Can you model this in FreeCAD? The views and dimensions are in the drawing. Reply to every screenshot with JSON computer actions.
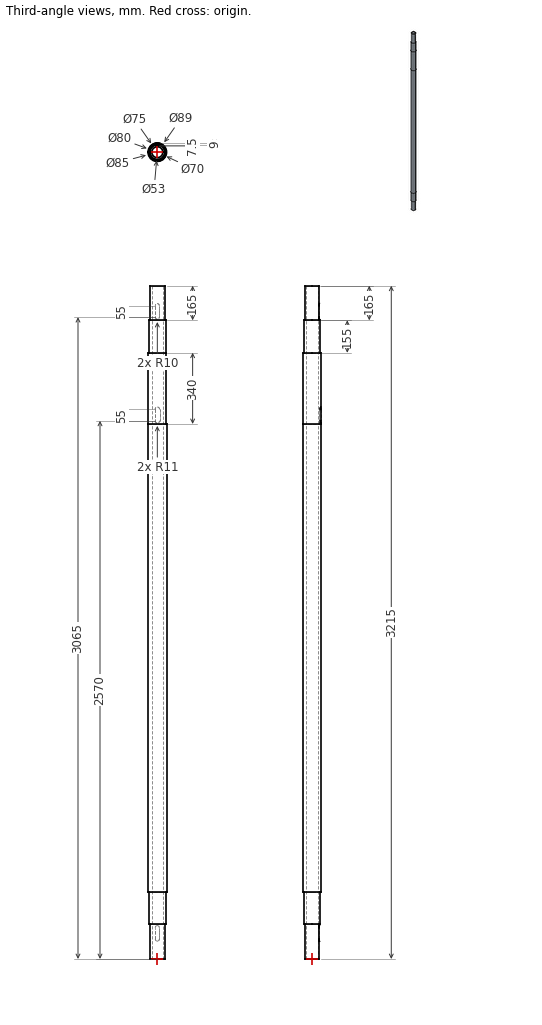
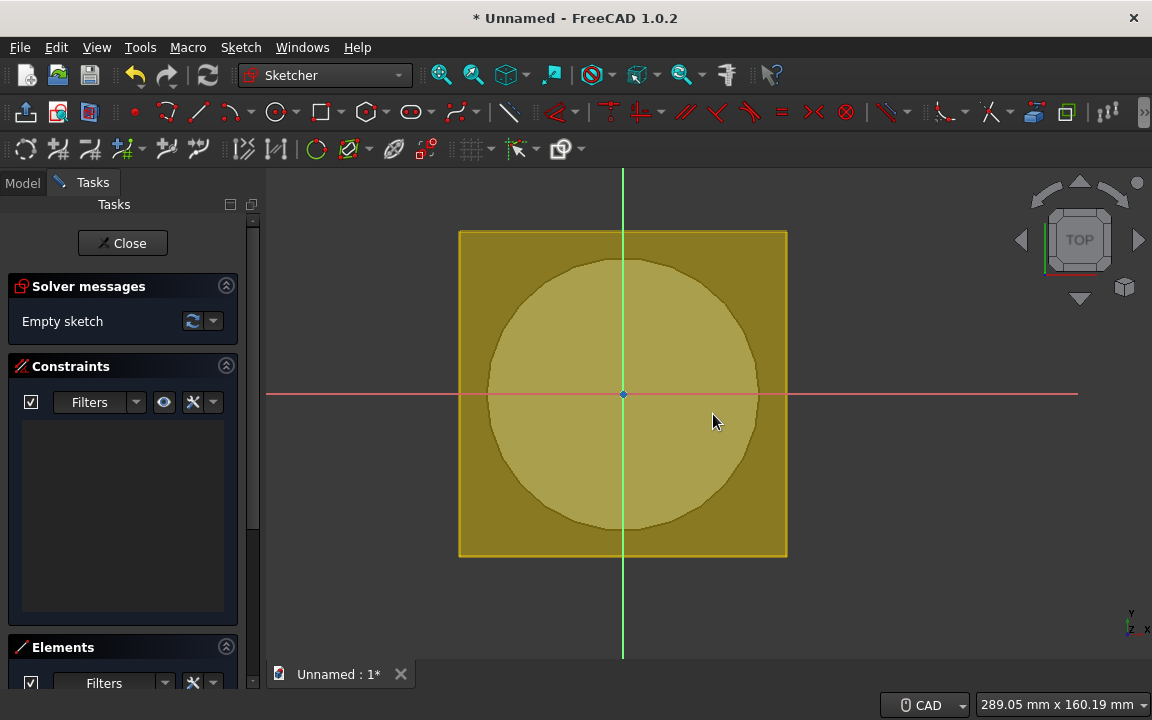
{"action": "left_click", "coordinate": [276, 112]}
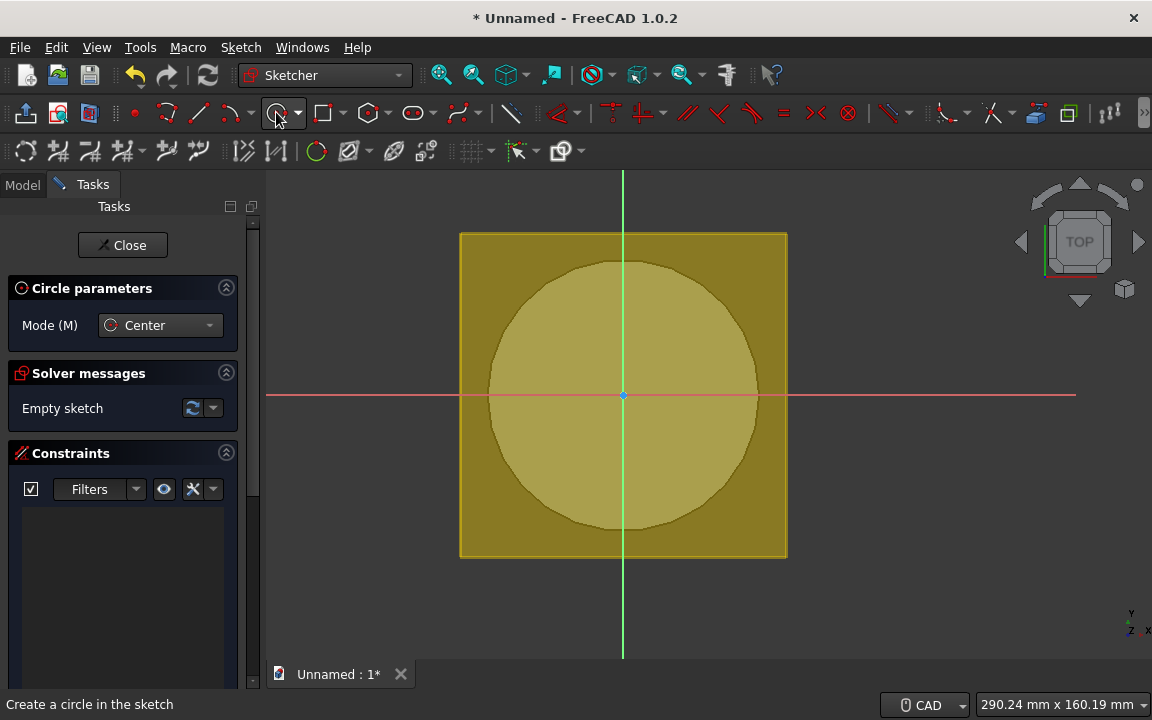
{"action": "left_click", "coordinate": [623, 395]}
{"action": "mouse_move", "coordinate": [719, 299]}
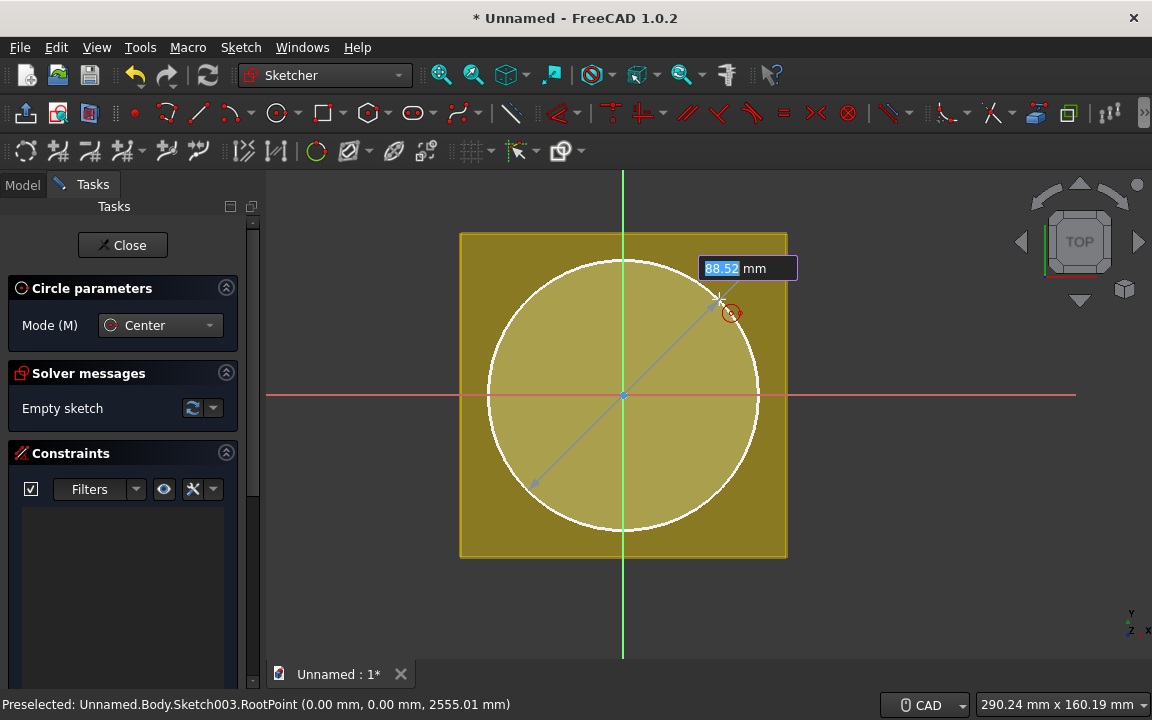
{"action": "type", "text": "89"}
{"action": "key", "text": "Return"}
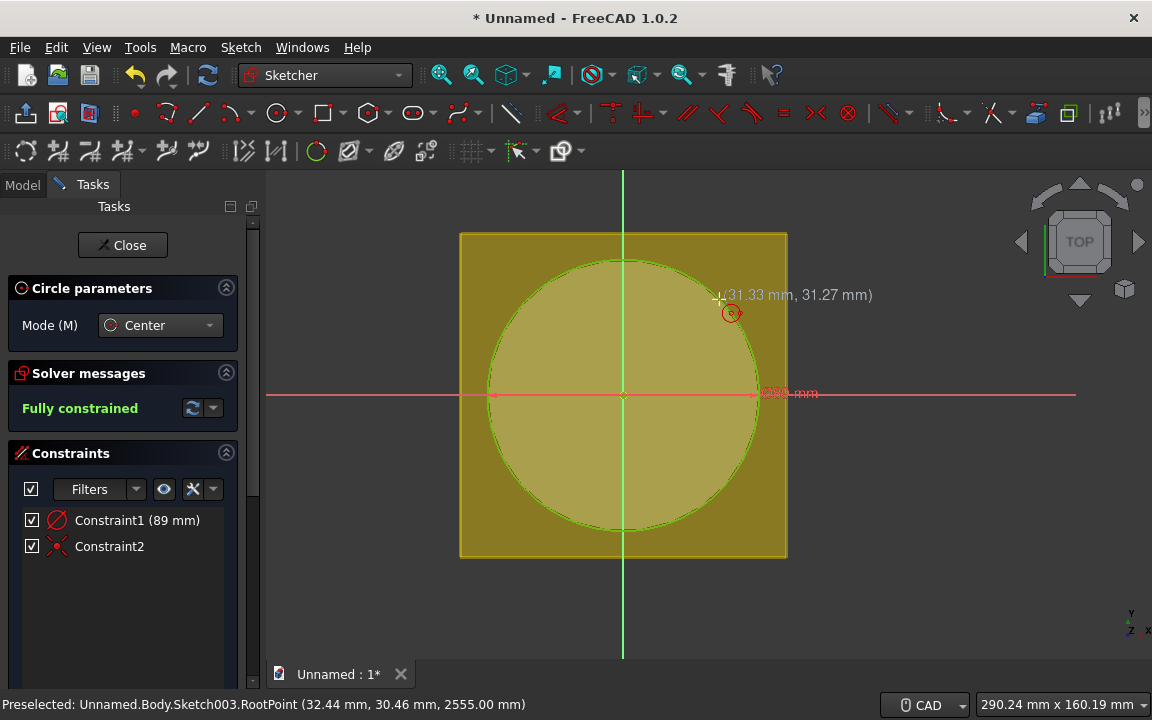
{"action": "left_click", "coordinate": [623, 395]}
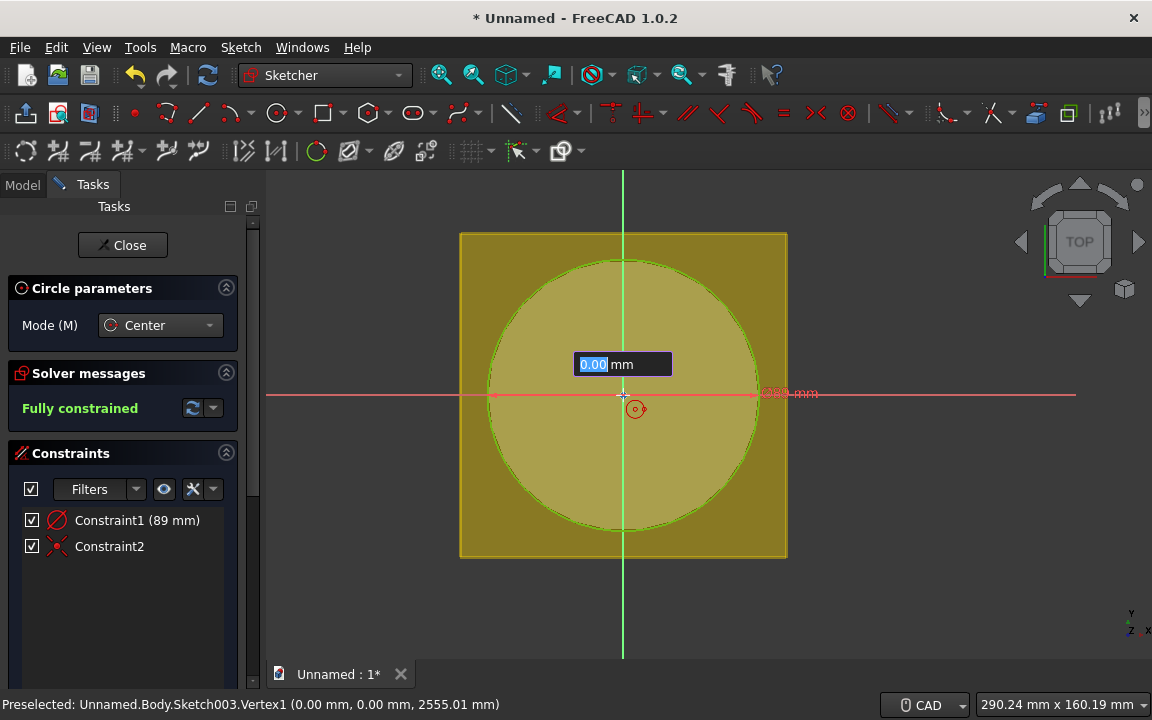
{"action": "scroll", "coordinate": [715, 304], "scroll_direction": "up", "scroll_amount": 5}
{"action": "mouse_move", "coordinate": [714, 303]}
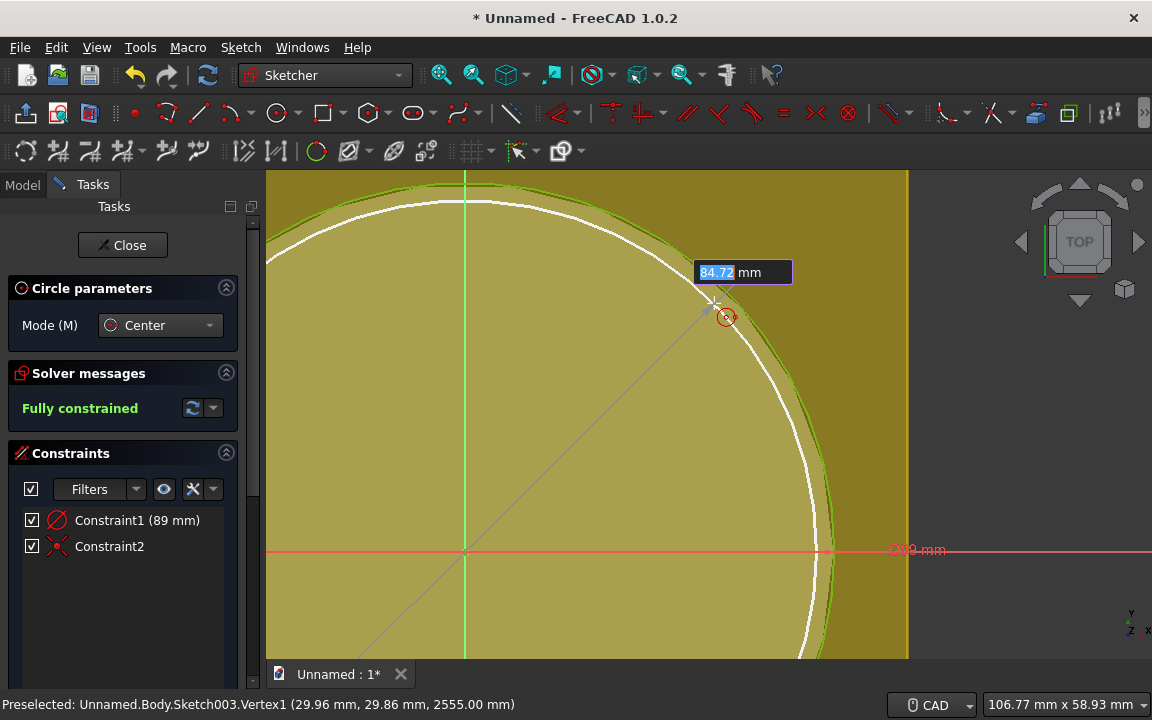
{"action": "type", "text": "85"}
{"action": "key", "text": "Return"}
{"action": "key", "text": "Escape"}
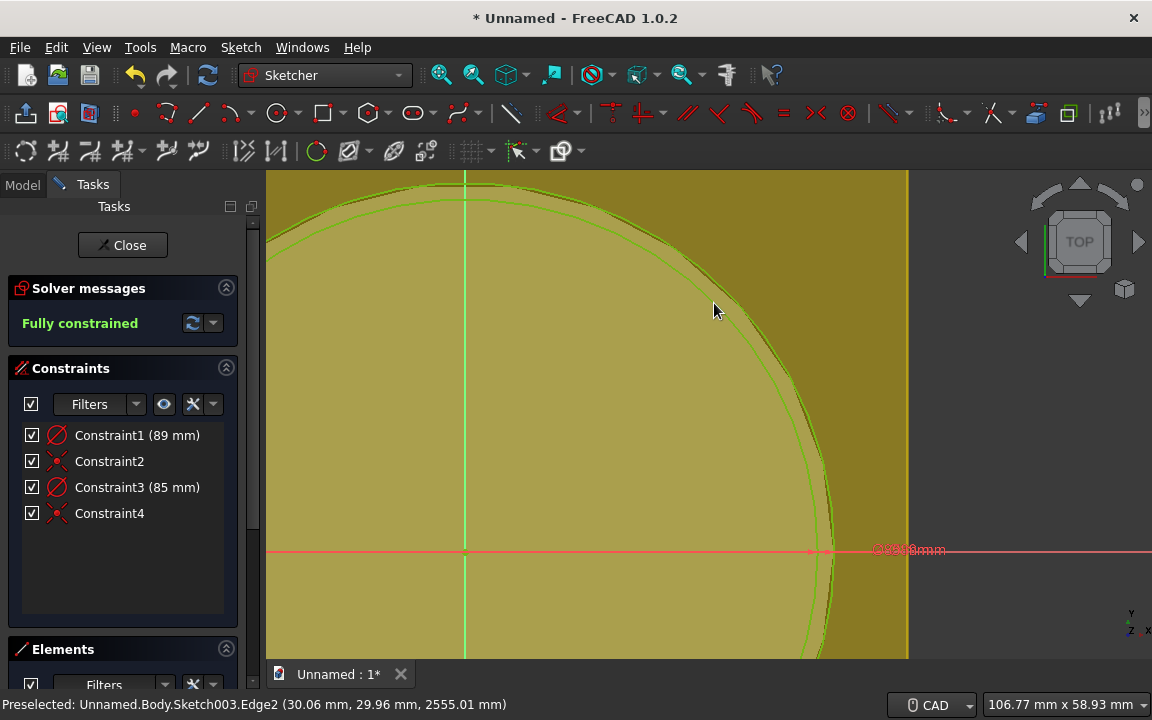
{"action": "left_click", "coordinate": [123, 245]}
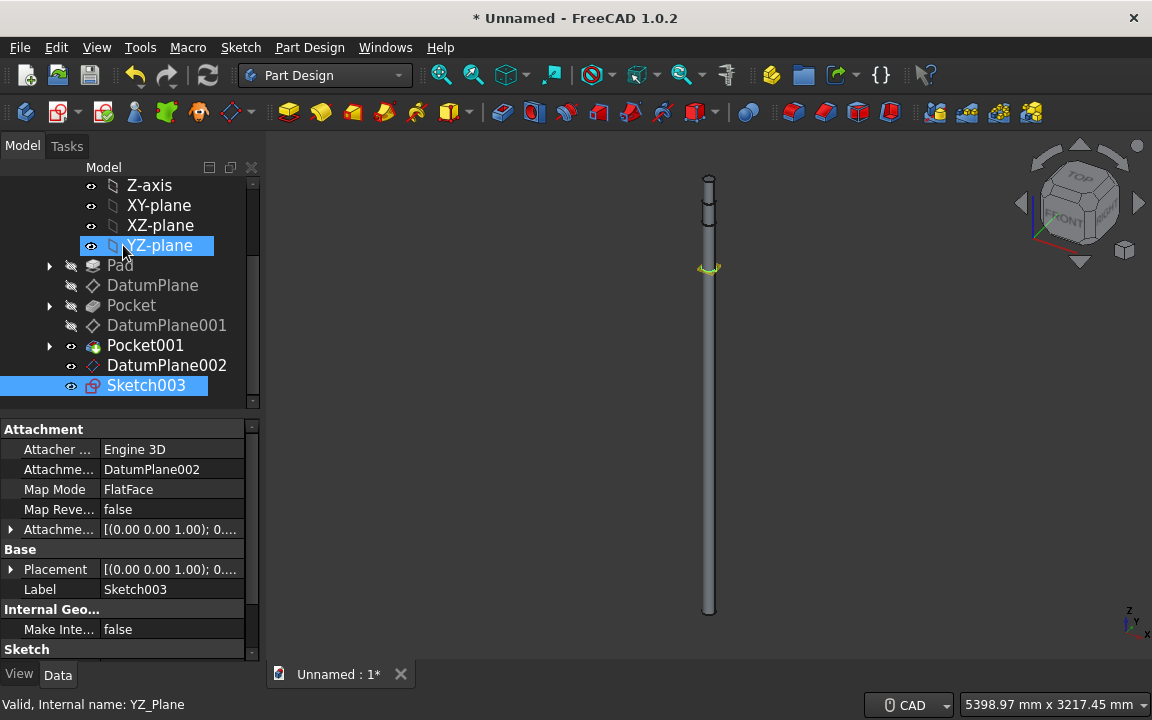
{"action": "left_click", "coordinate": [504, 112]}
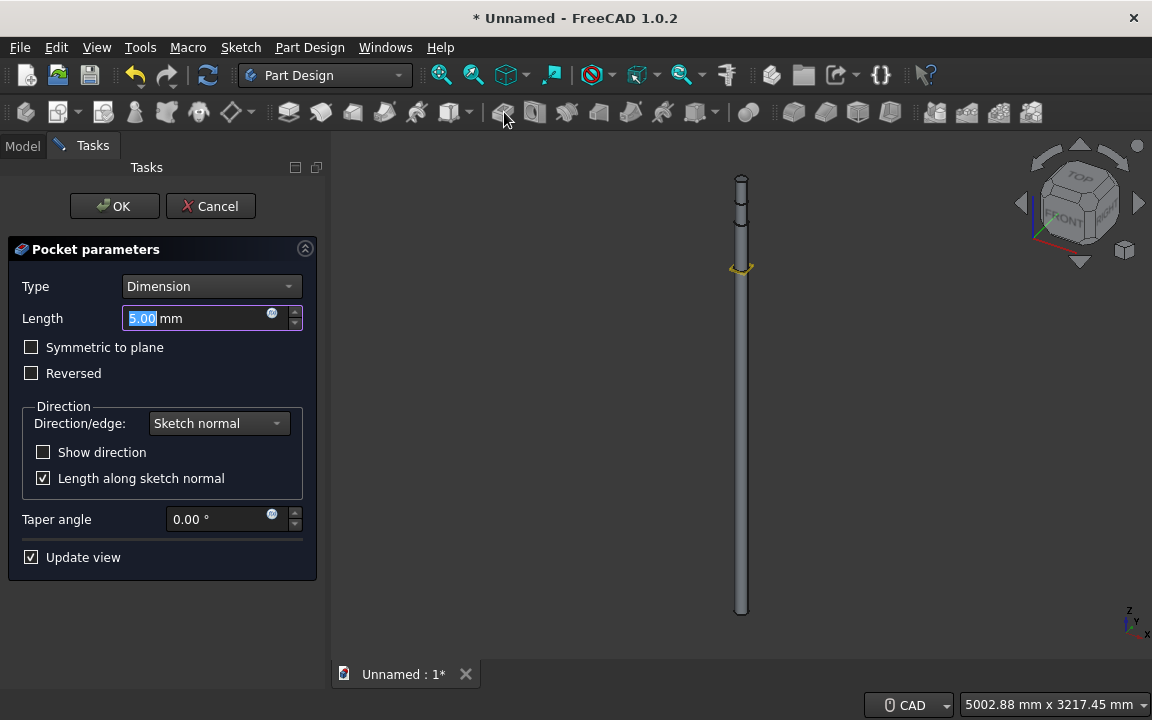
{"action": "type", "text": "340"}
{"action": "key", "text": "Tab"}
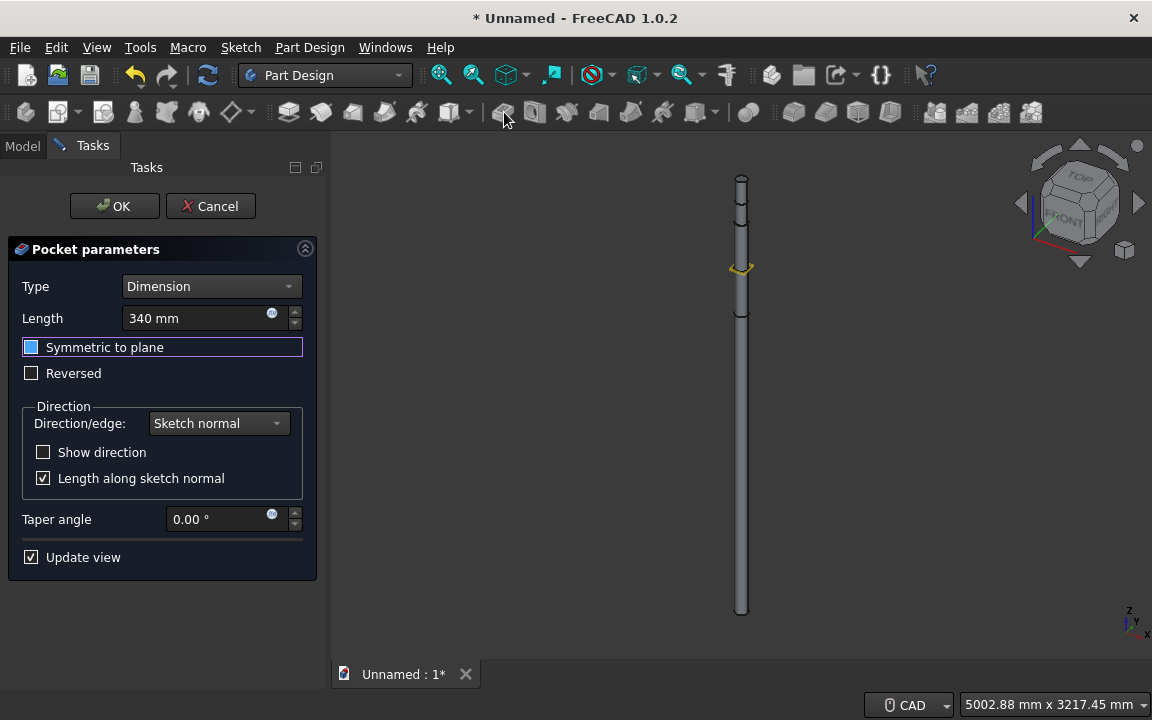
{"action": "left_click", "coordinate": [30, 373]}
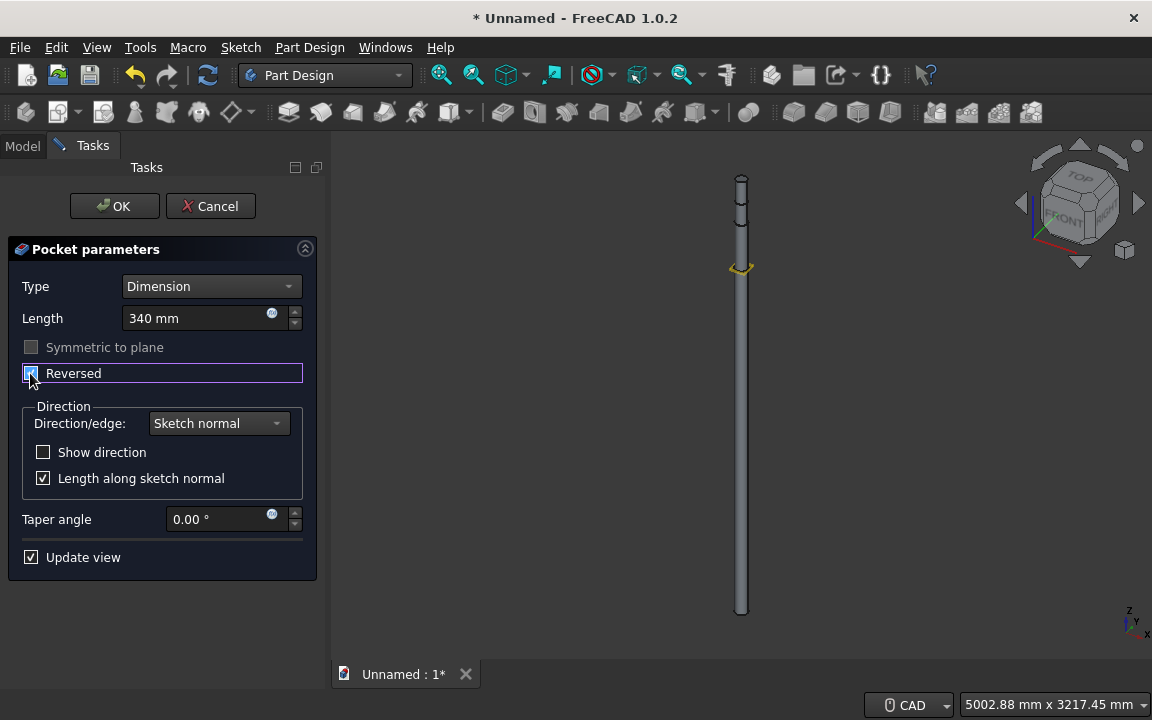
{"action": "left_click", "coordinate": [115, 206]}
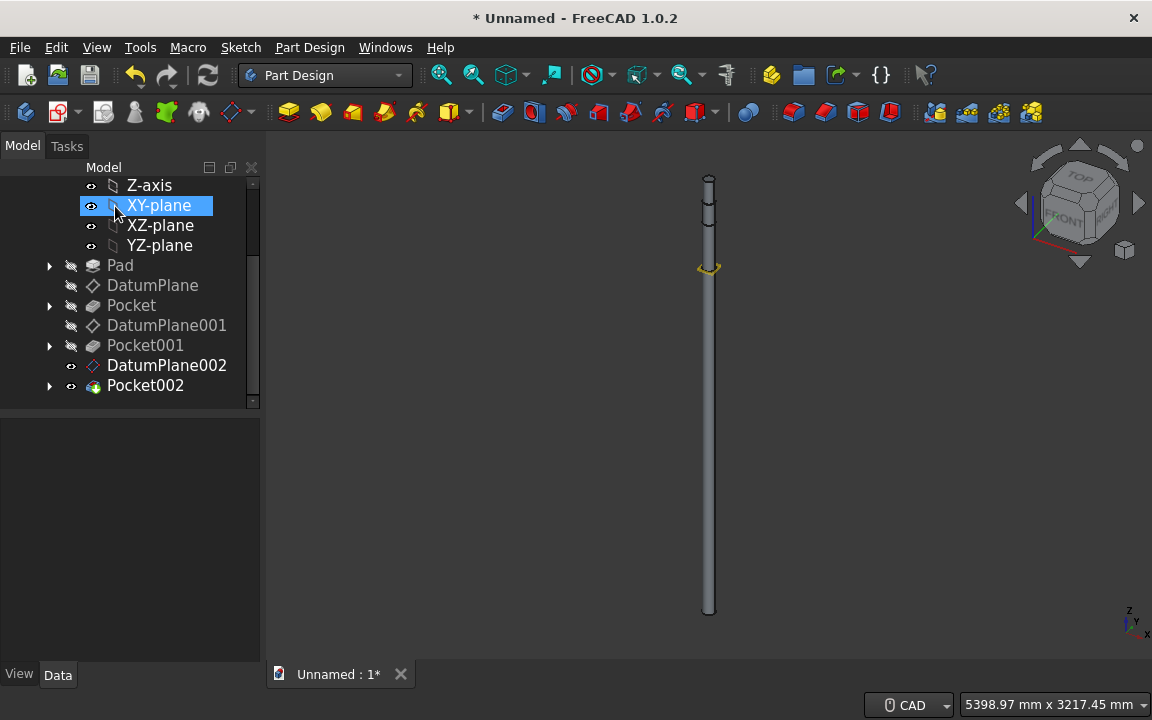
{"action": "left_click", "coordinate": [116, 366]}
{"action": "key", "text": "space"}